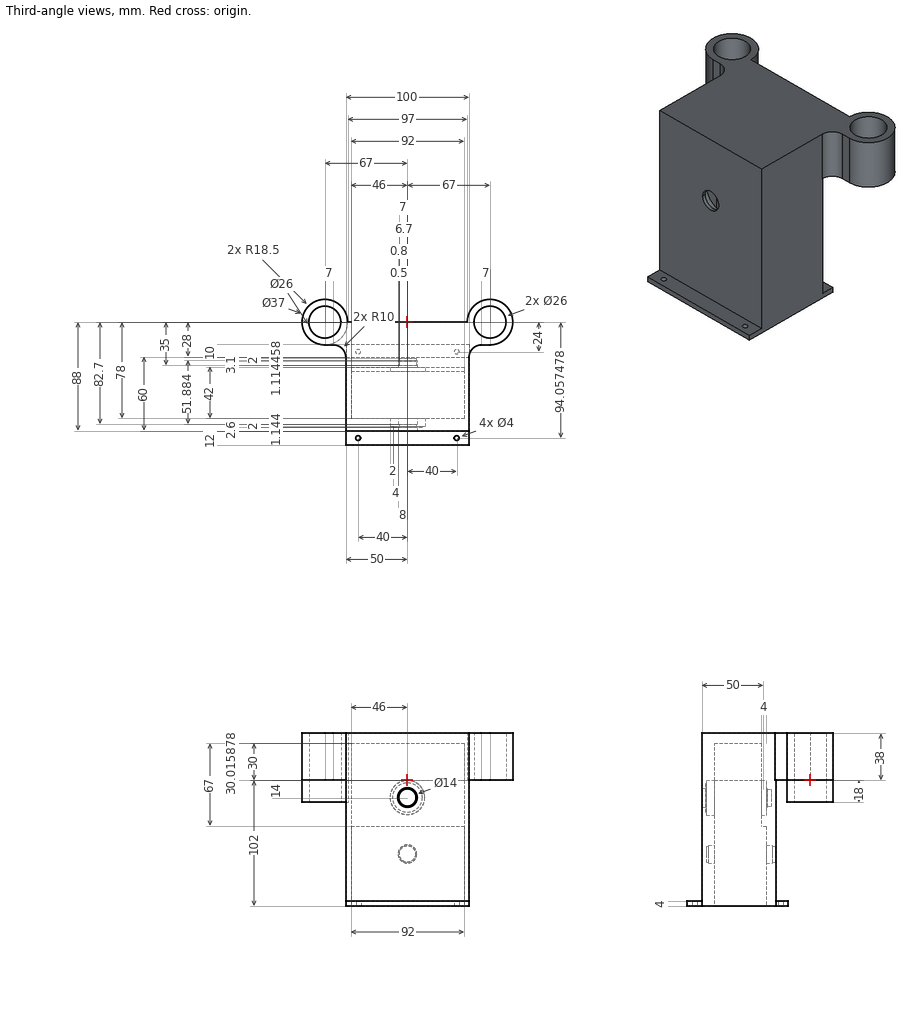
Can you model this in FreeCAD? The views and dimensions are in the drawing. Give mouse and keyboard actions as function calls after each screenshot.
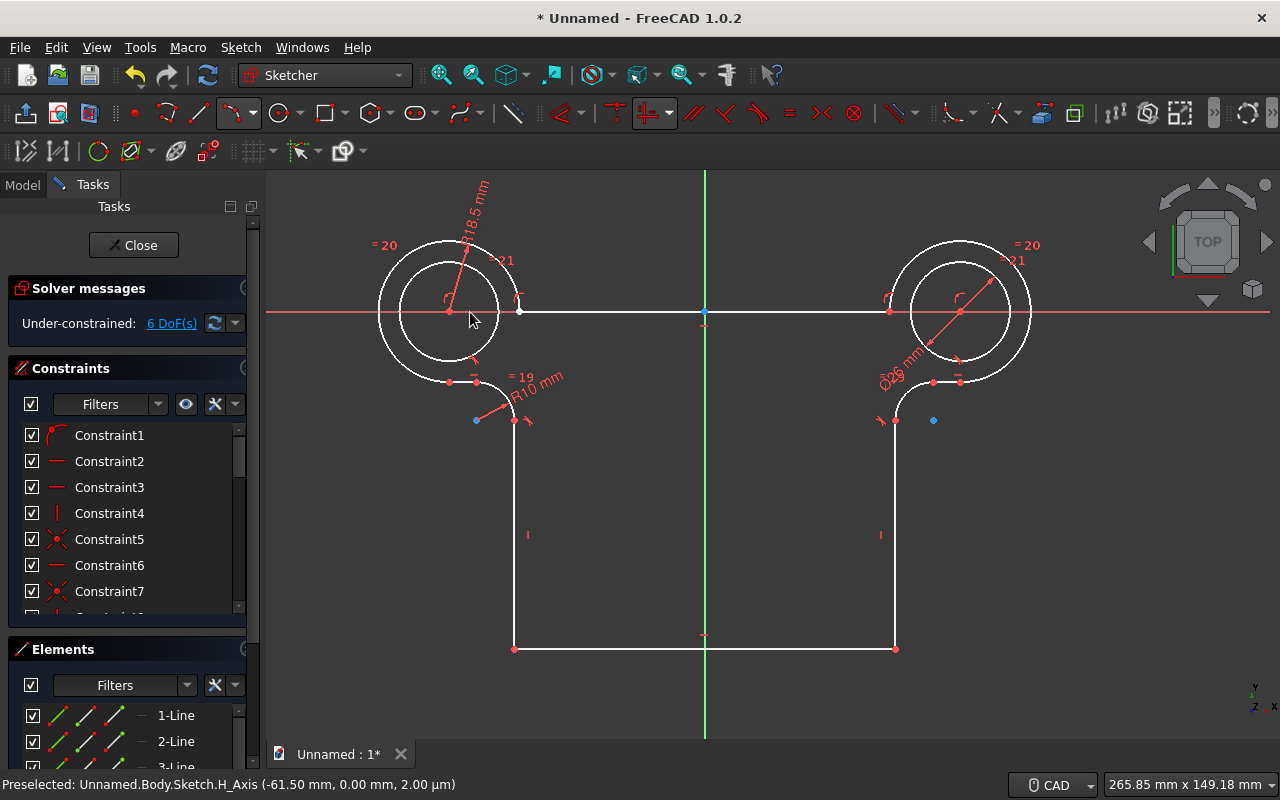
key(d)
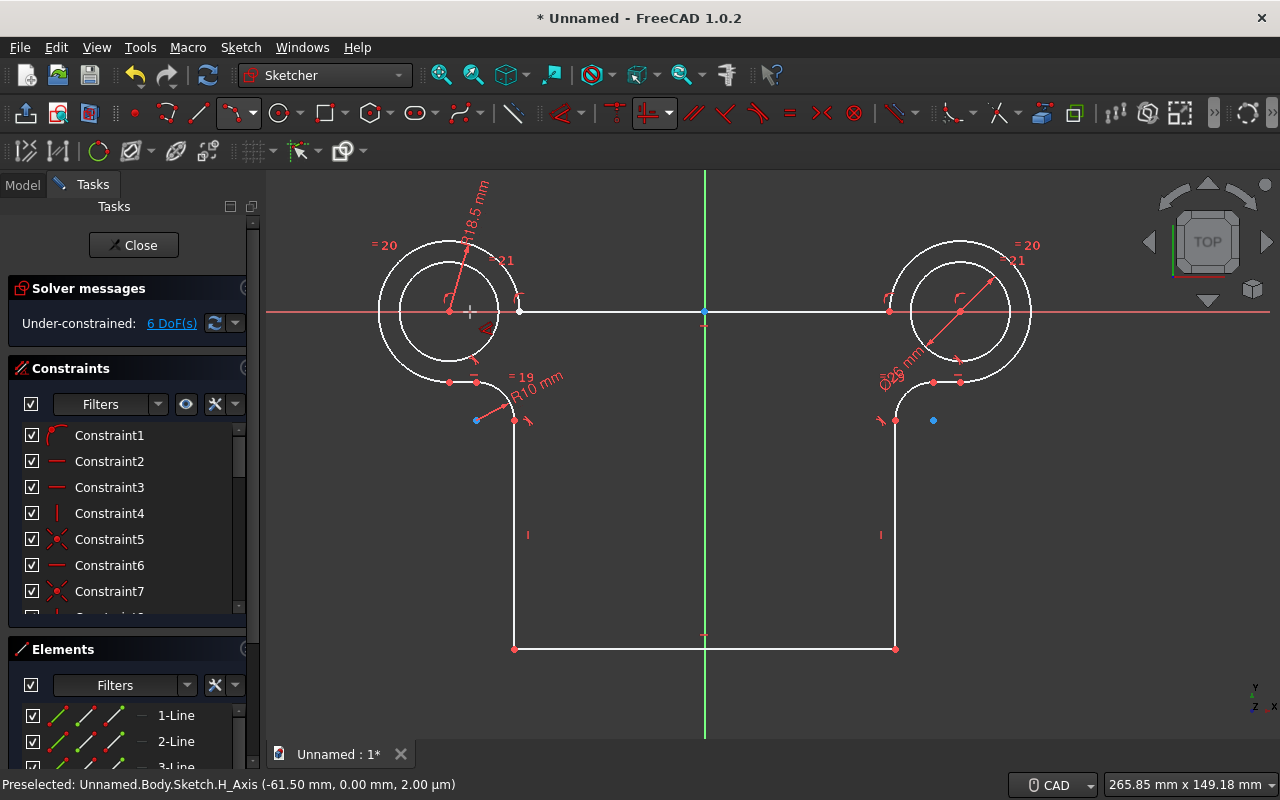
scroll(460, 382, up, 2)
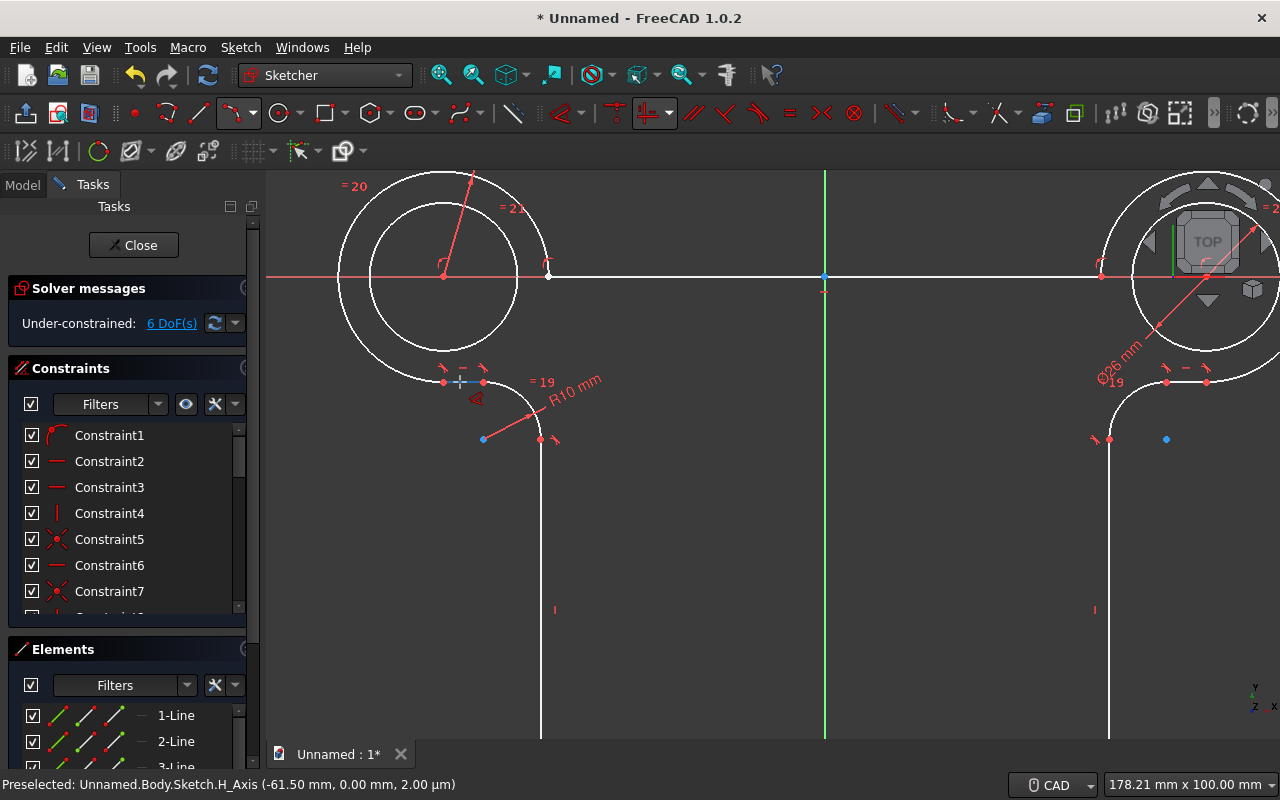
click(460, 382)
click(464, 416)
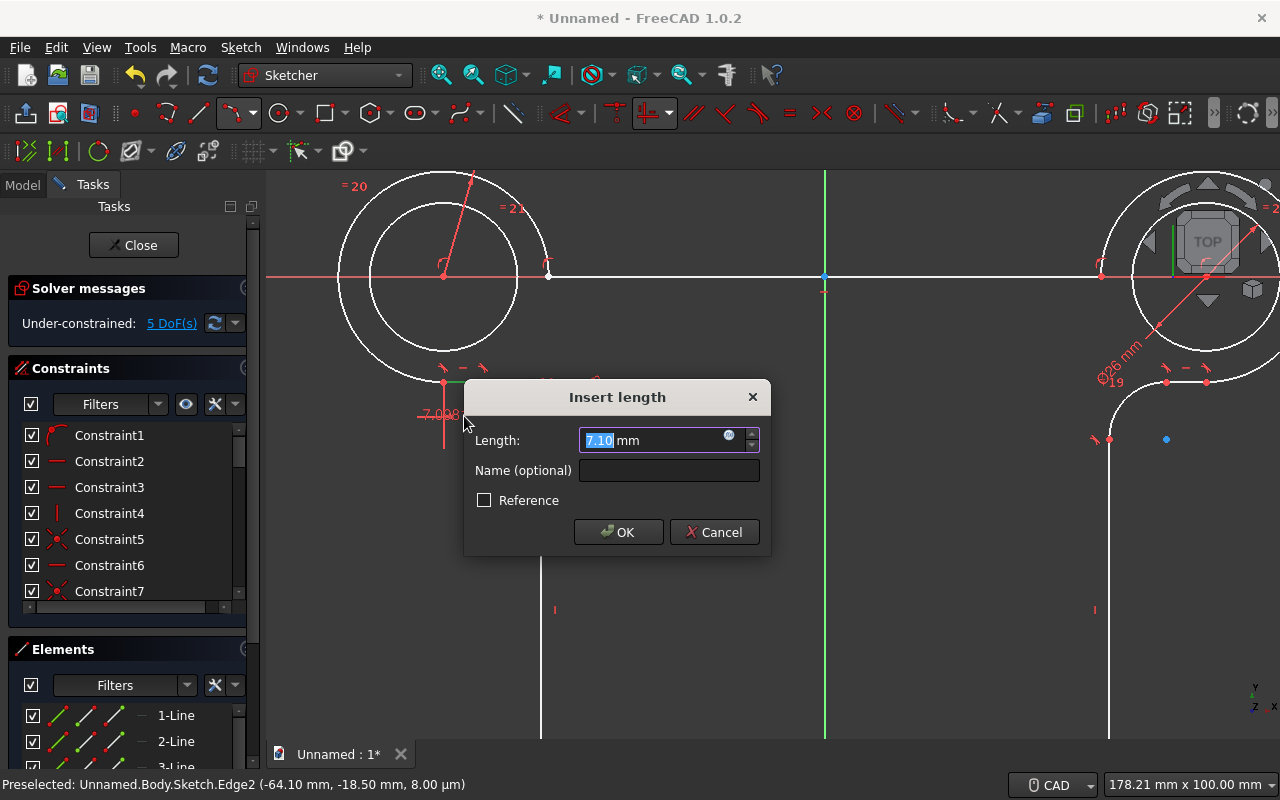
text(7)
key(Return)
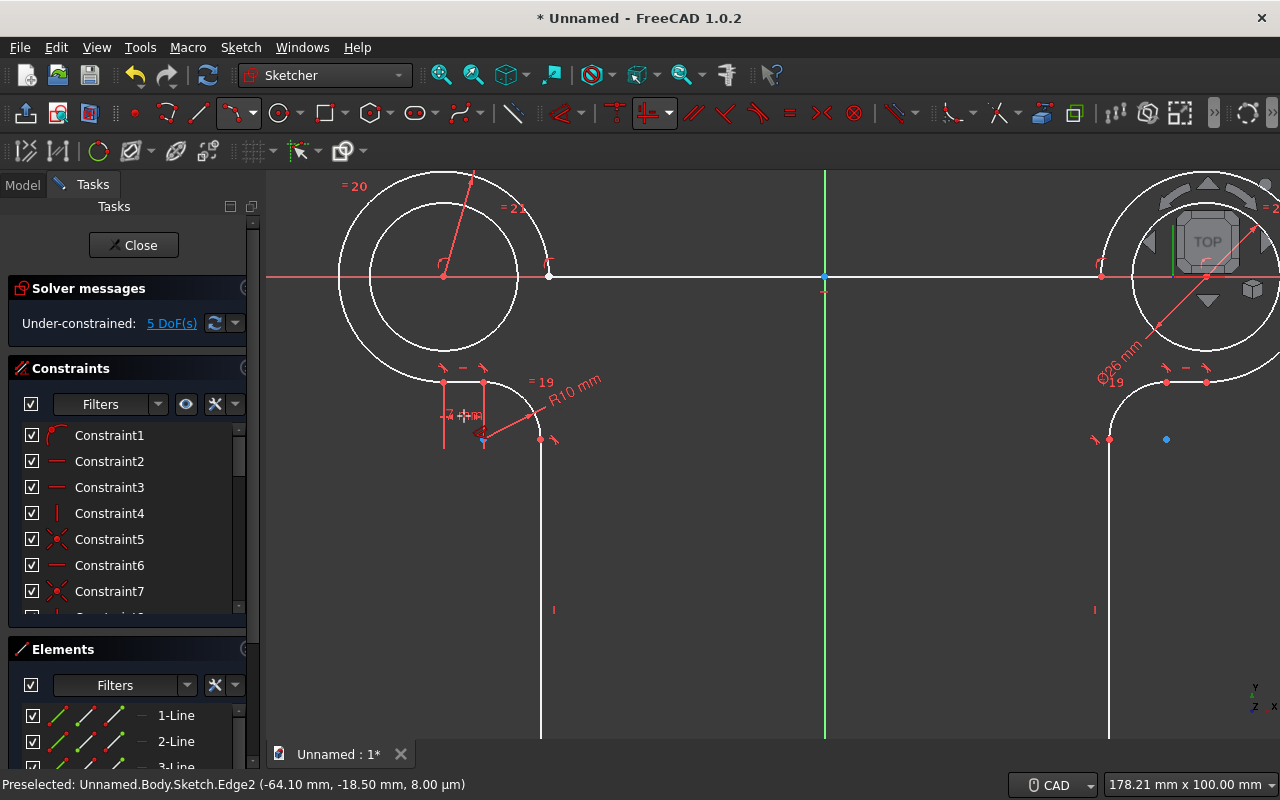
scroll(460, 382, down, 2)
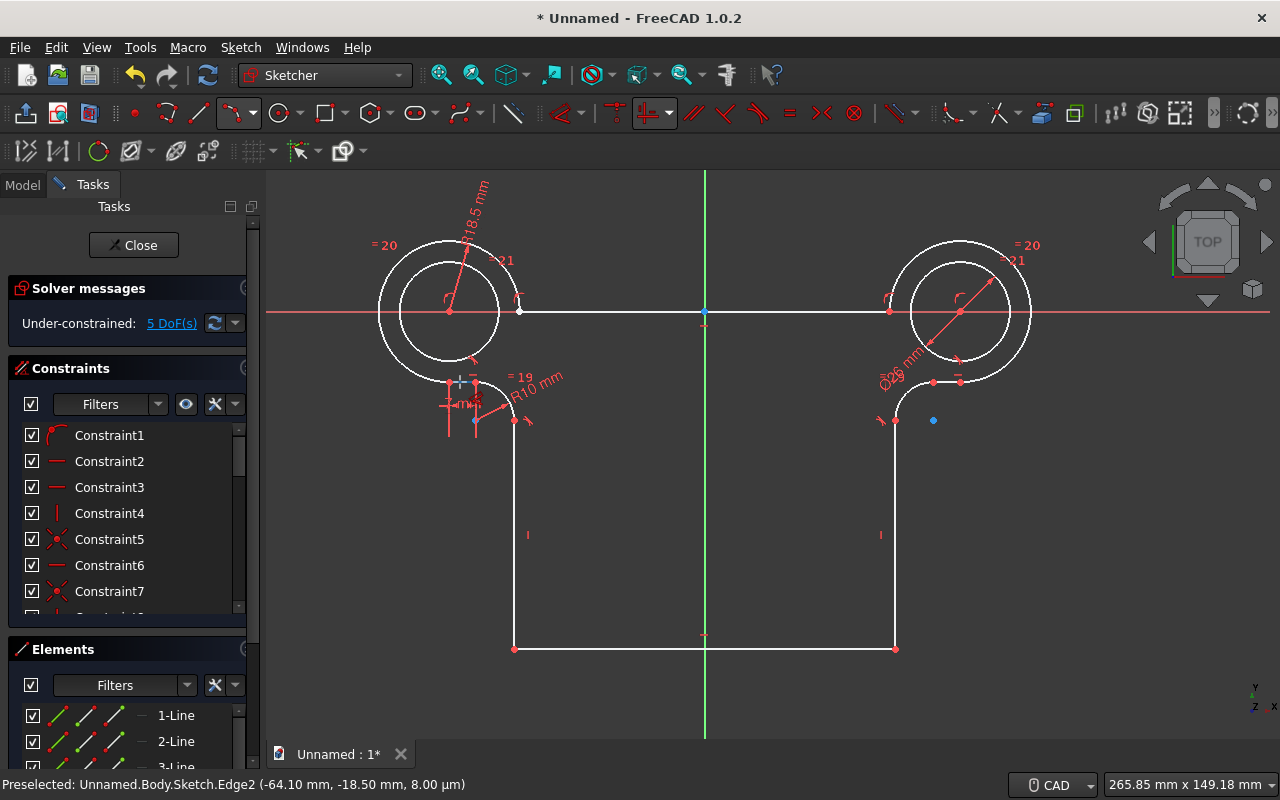
scroll(942, 382, up, 3)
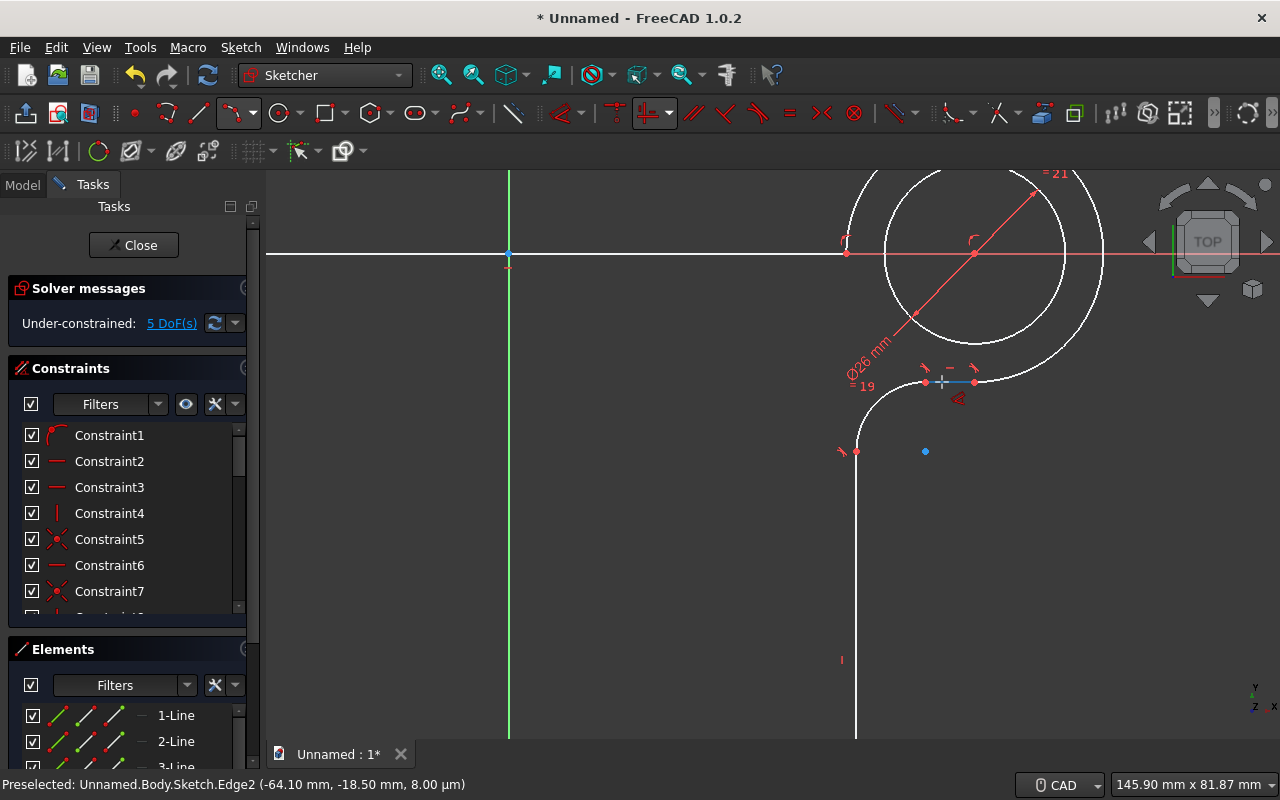
click(941, 382)
click(950, 416)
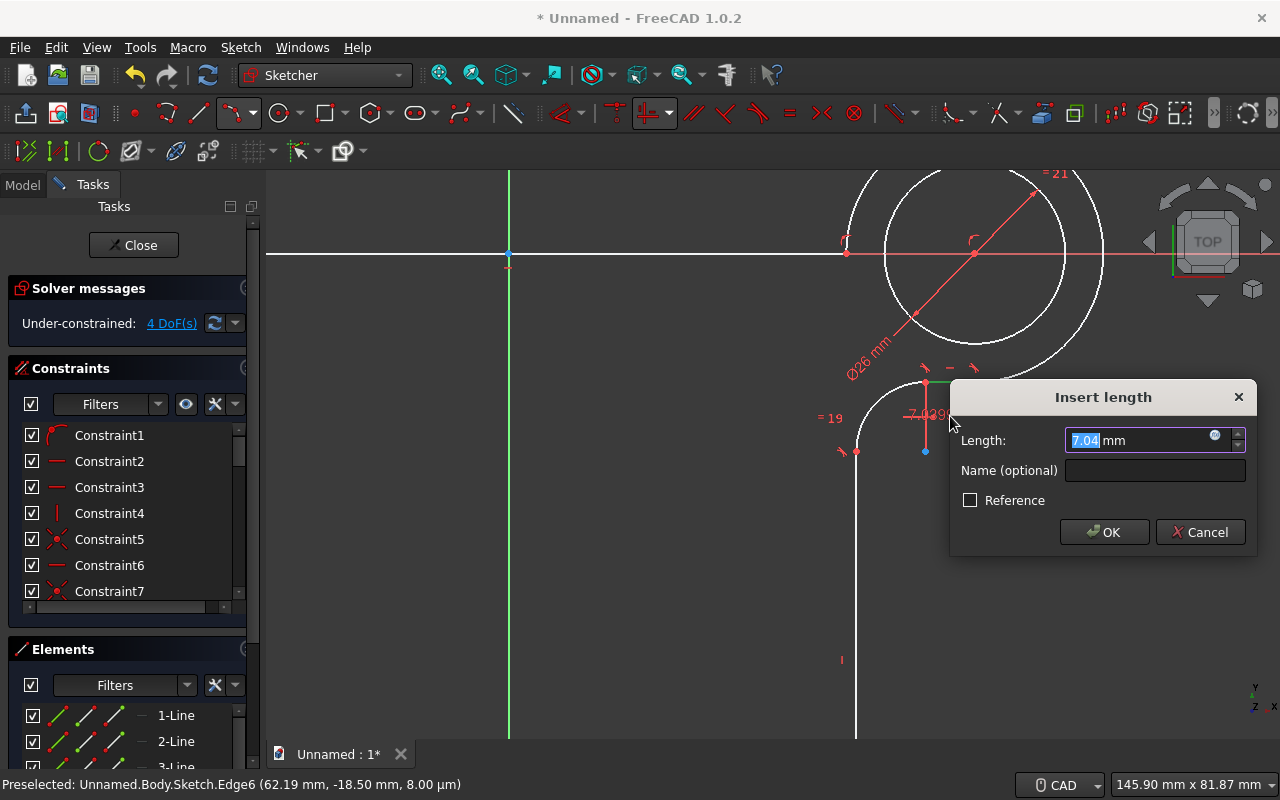
text(7)
key(Return)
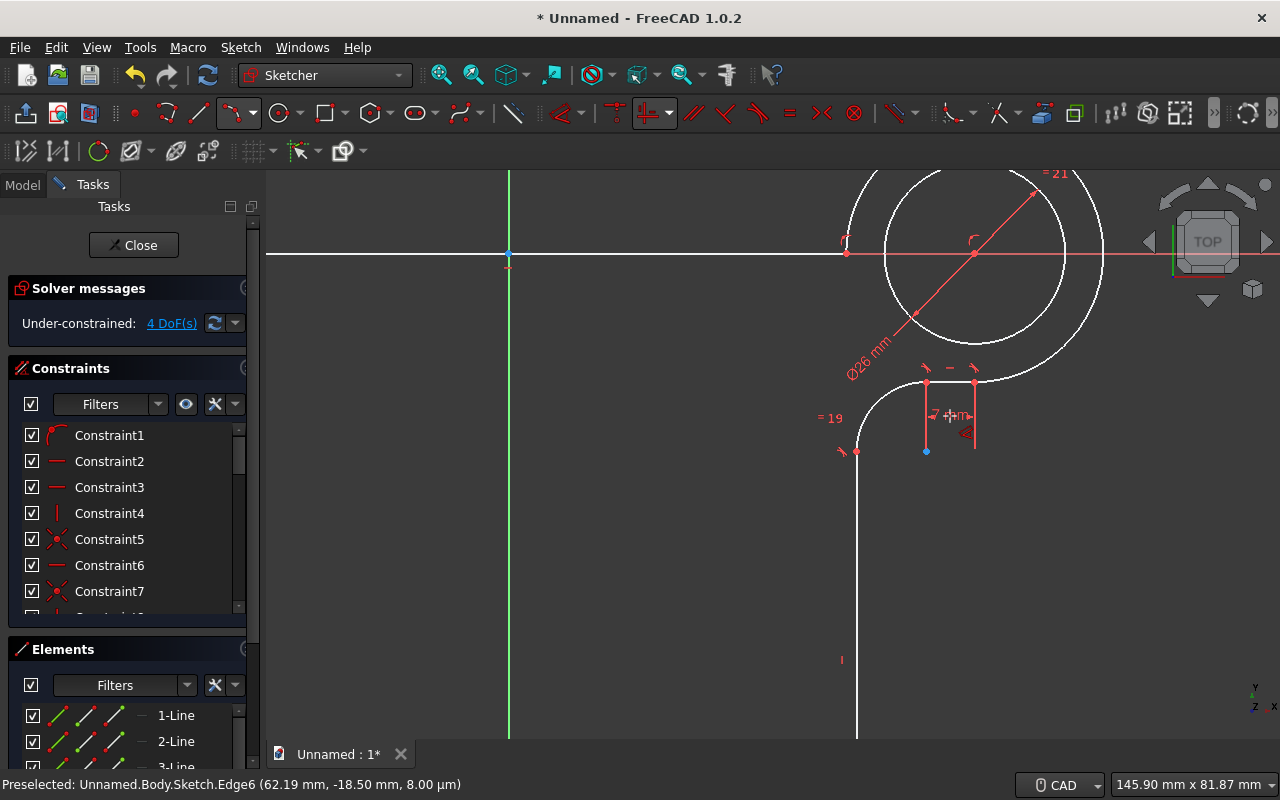
click(644, 254)
click(570, 220)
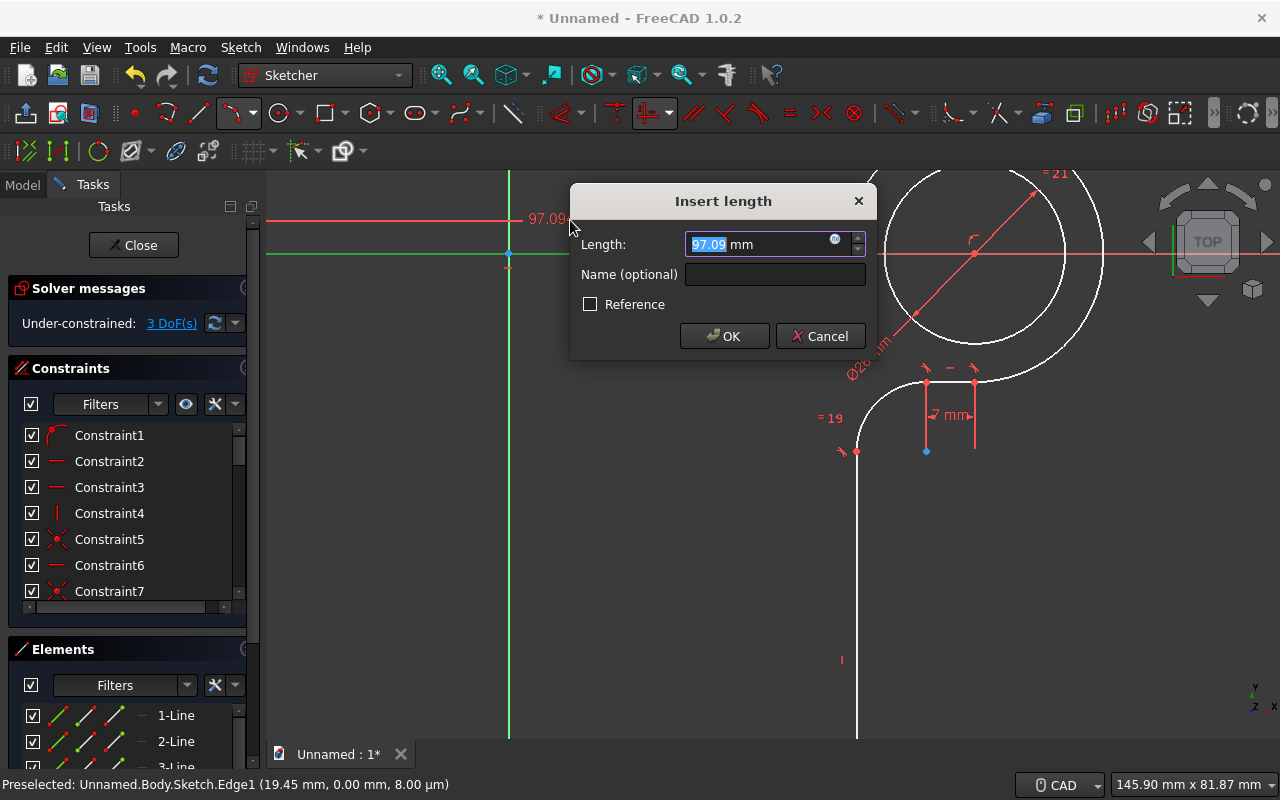
text(97)
key(Return)